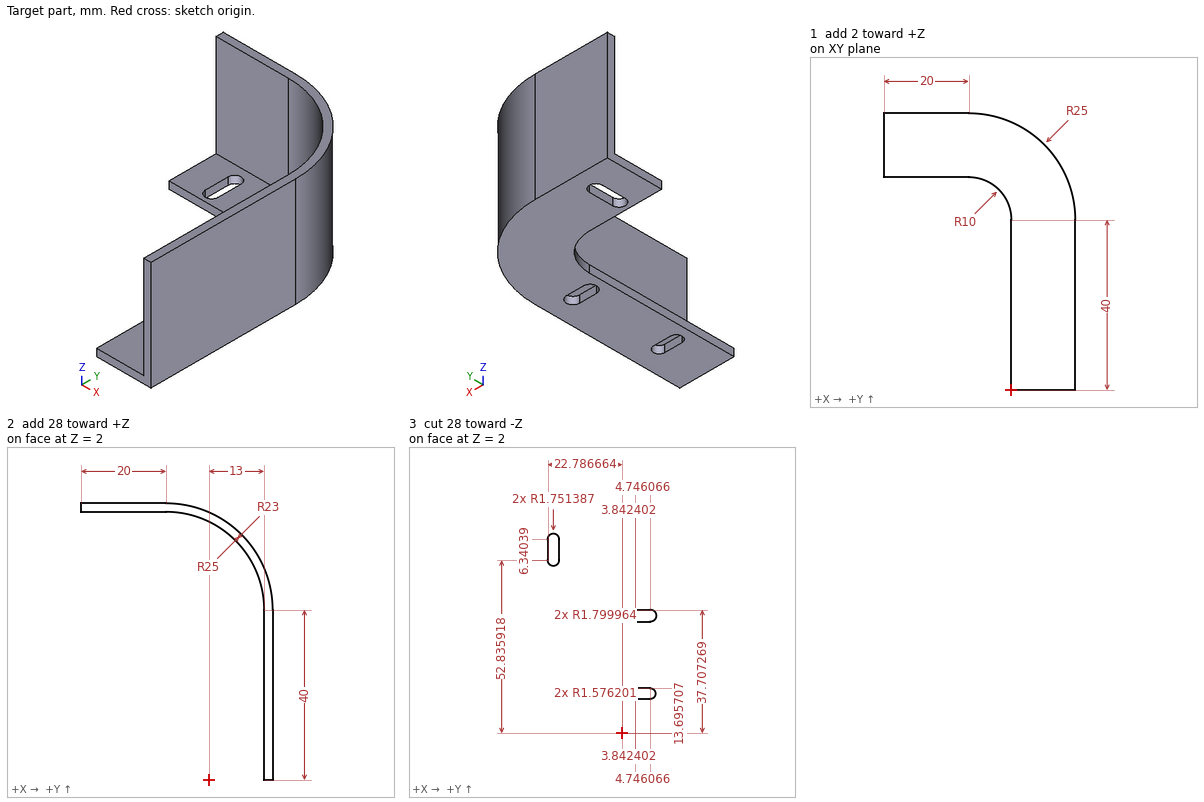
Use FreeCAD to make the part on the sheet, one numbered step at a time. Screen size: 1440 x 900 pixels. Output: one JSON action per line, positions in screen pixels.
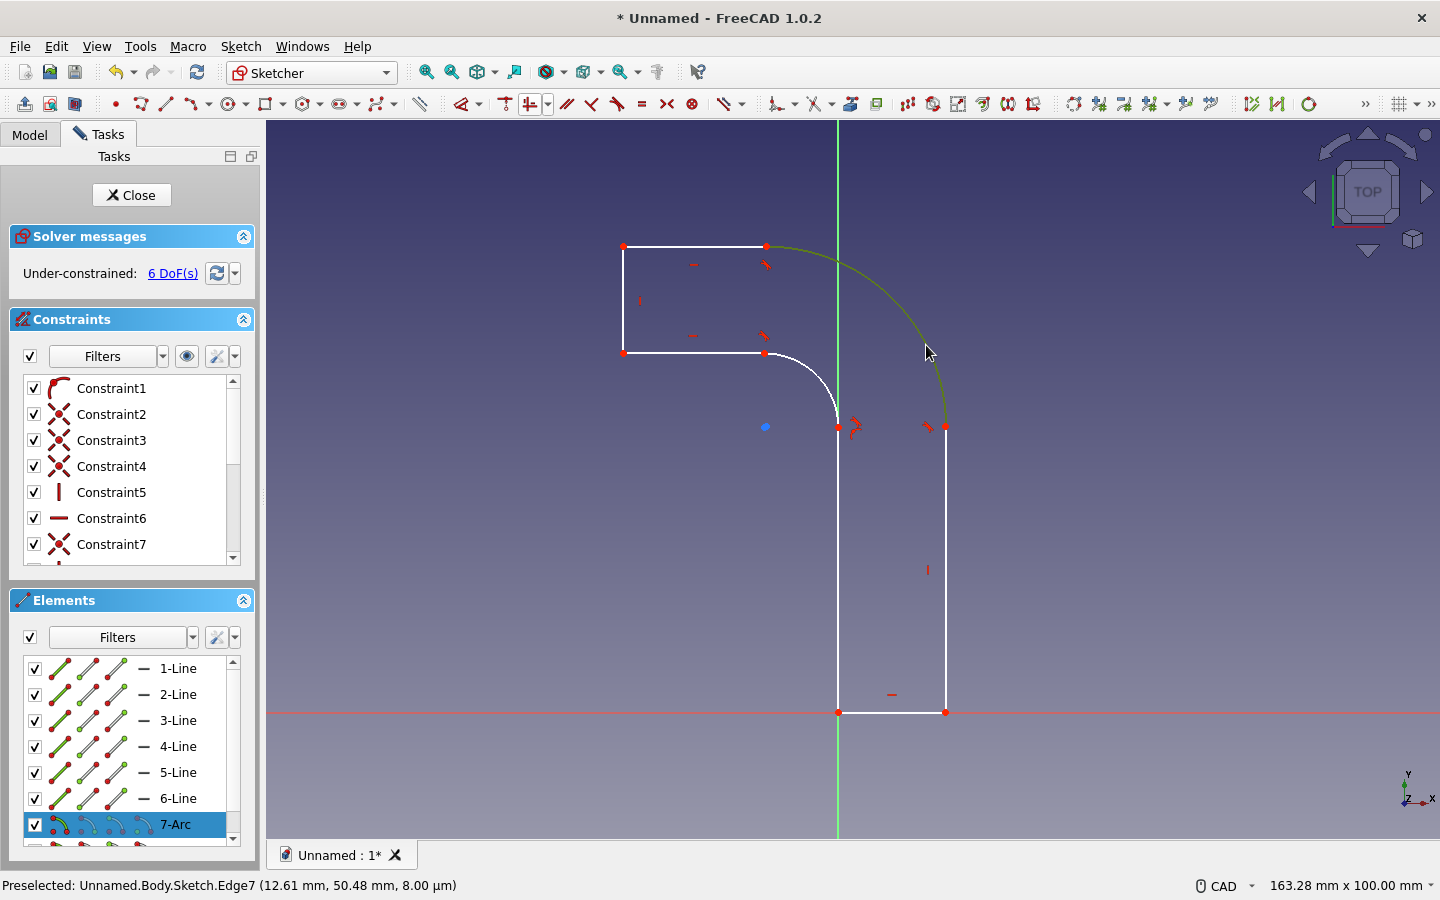
{"action": "left_click", "coordinate": [798, 362]}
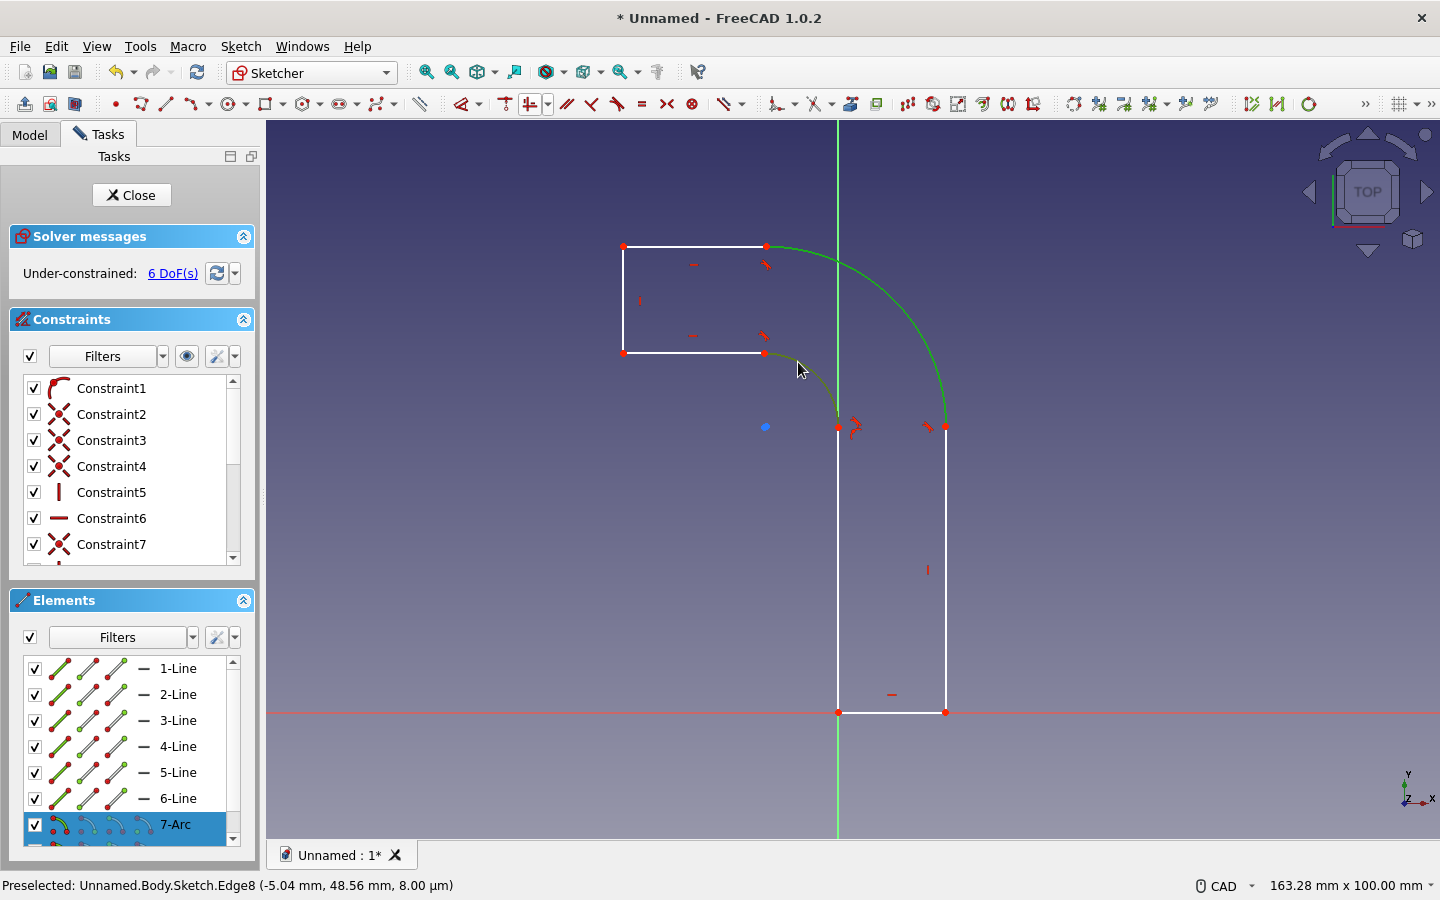
{"action": "left_click", "coordinate": [505, 104]}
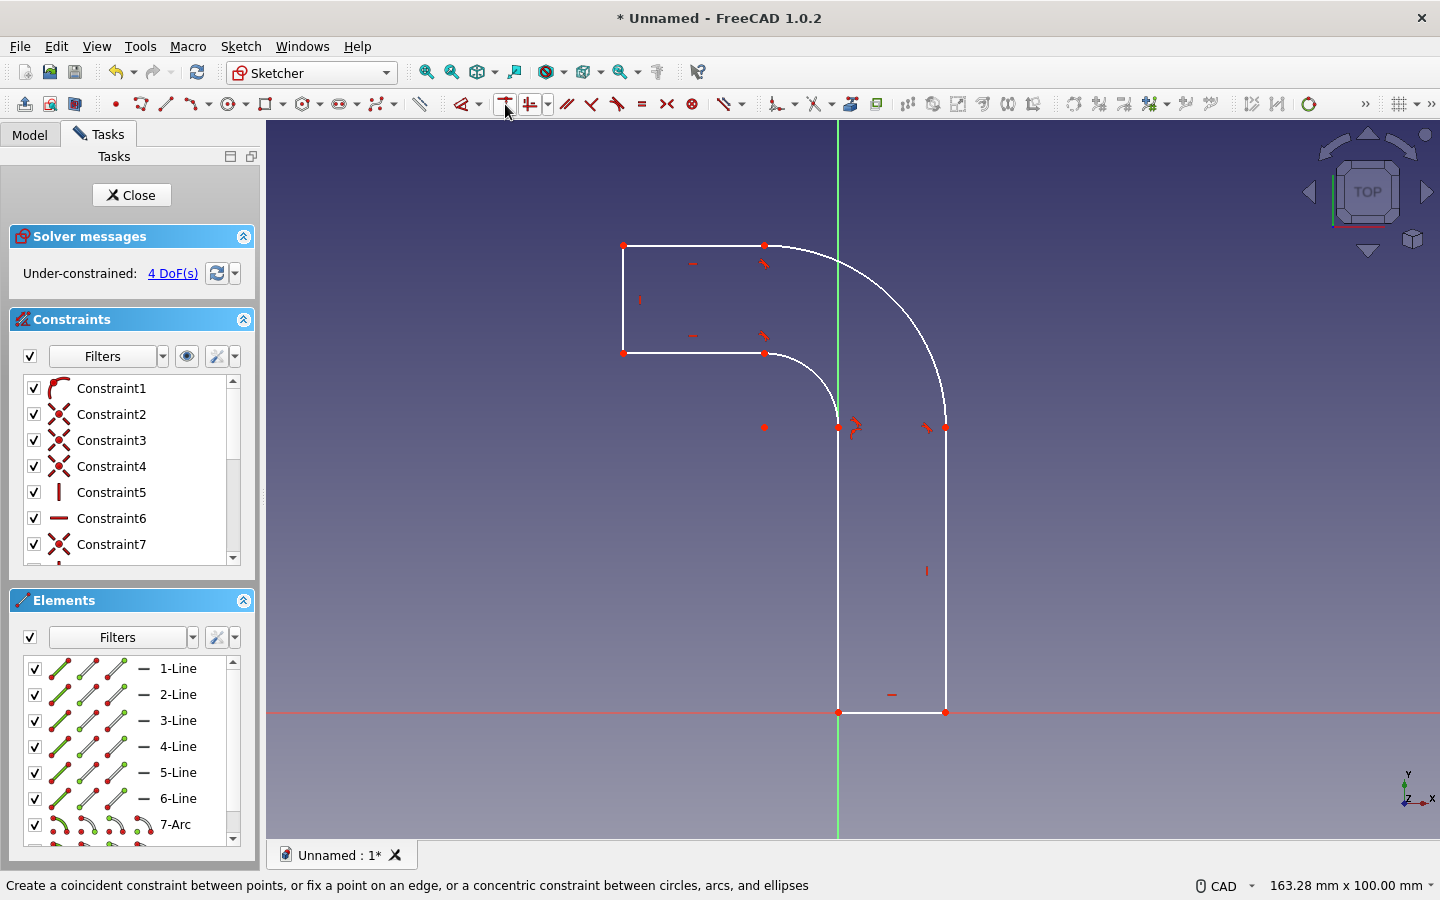
{"action": "left_click", "coordinate": [460, 104]}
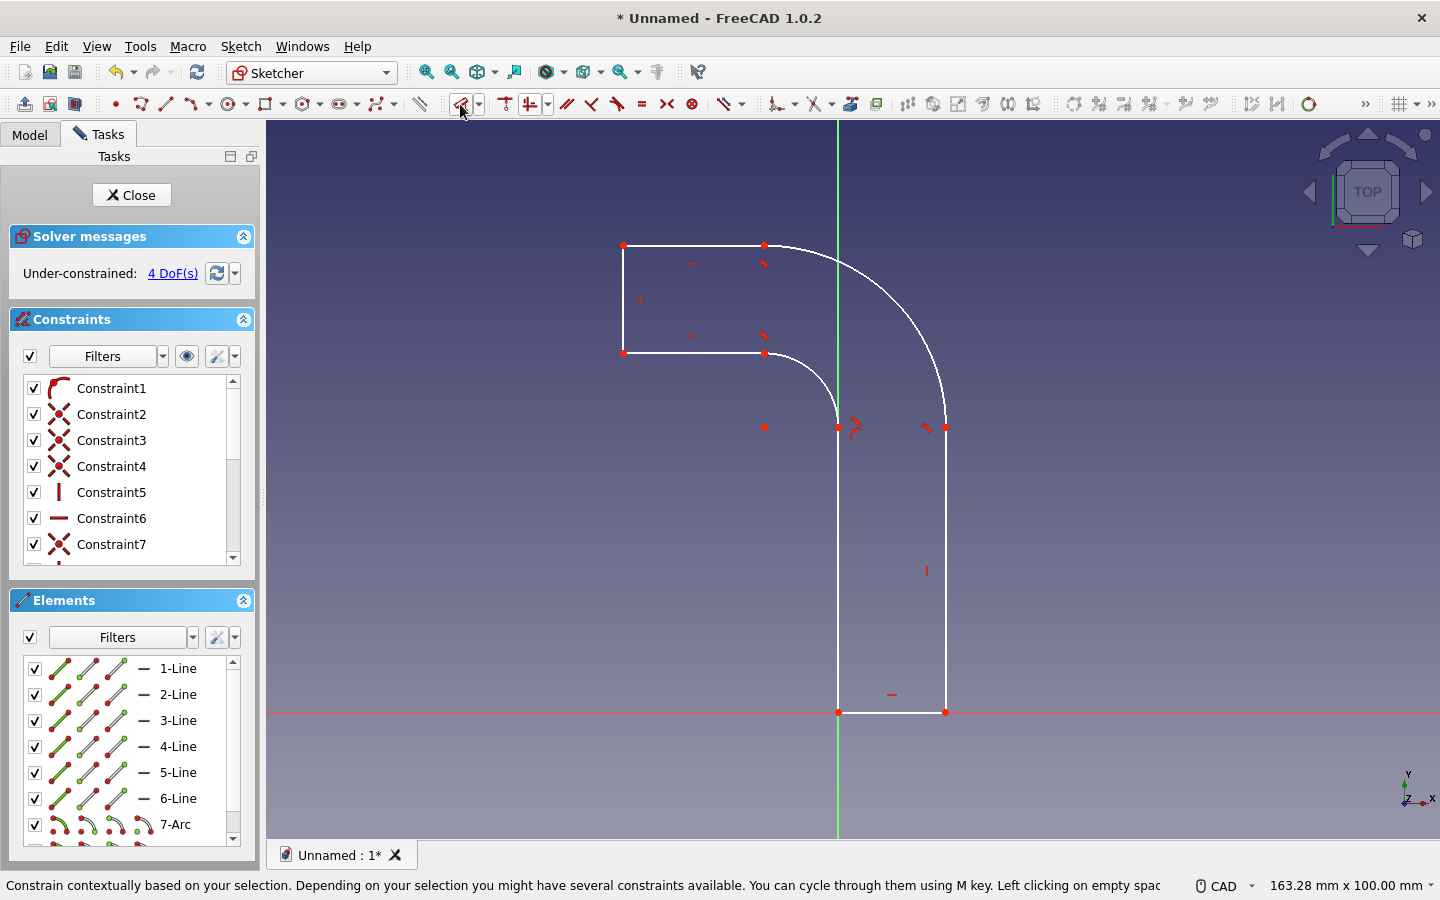
{"action": "left_click", "coordinate": [926, 345]}
{"action": "left_click", "coordinate": [955, 330]}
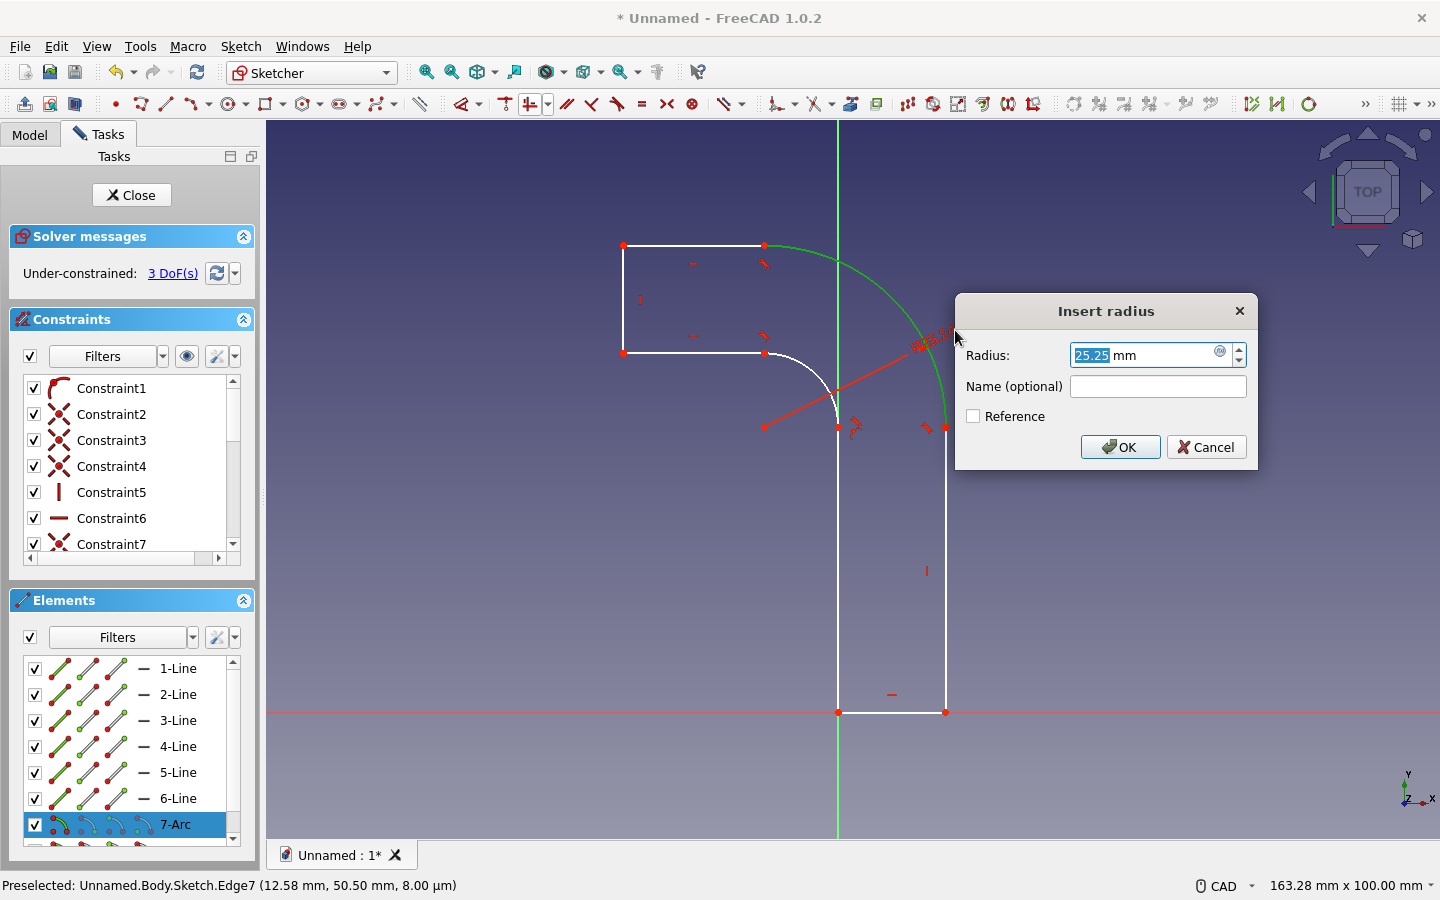
{"action": "type", "text": "25"}
{"action": "key", "text": "Return"}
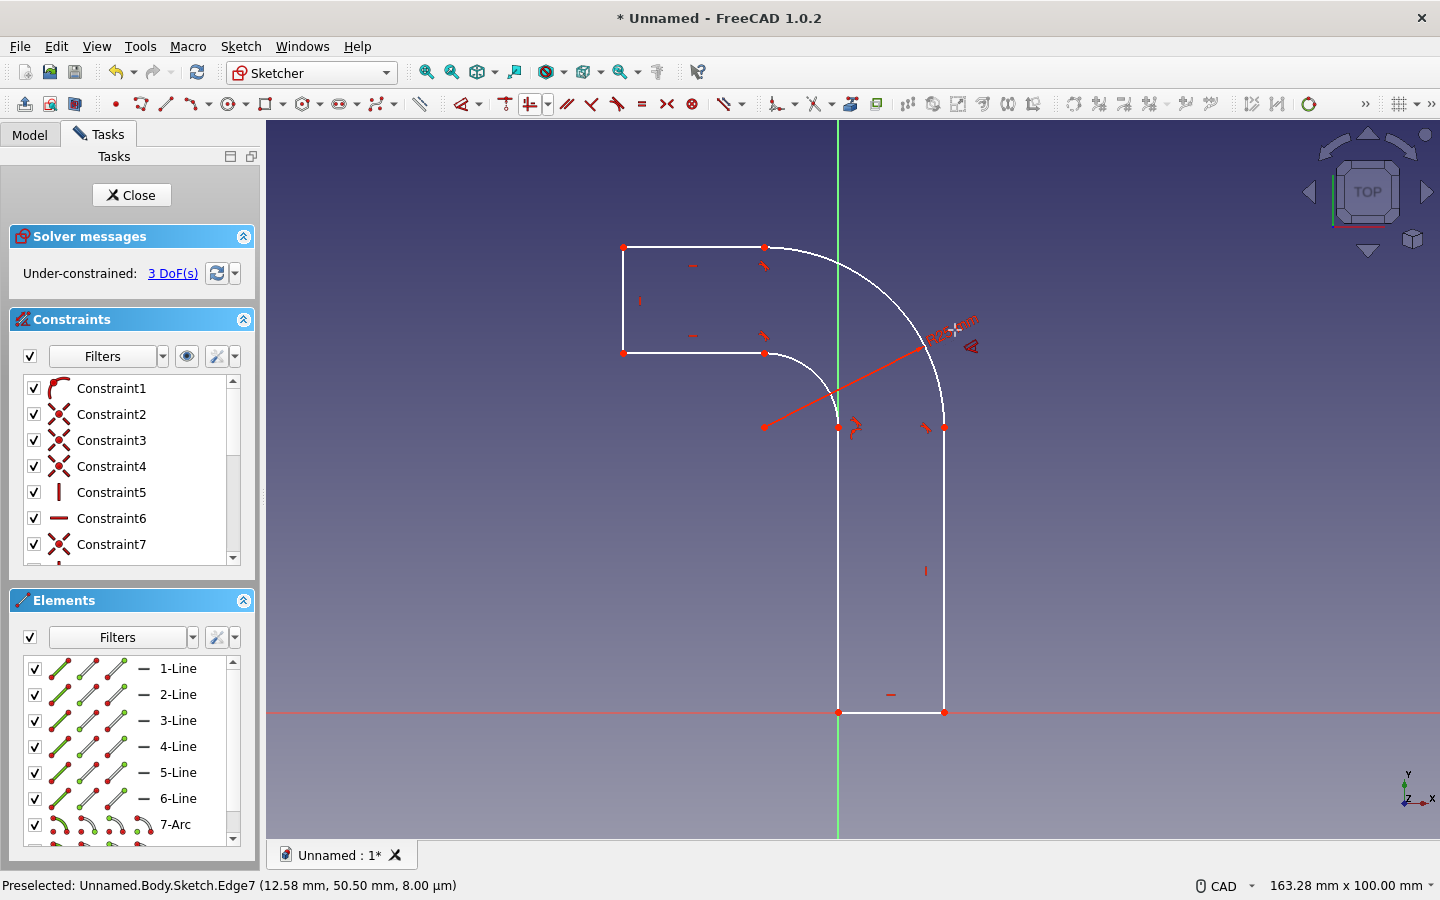
{"action": "left_click", "coordinate": [798, 361]}
{"action": "left_click", "coordinate": [812, 332]}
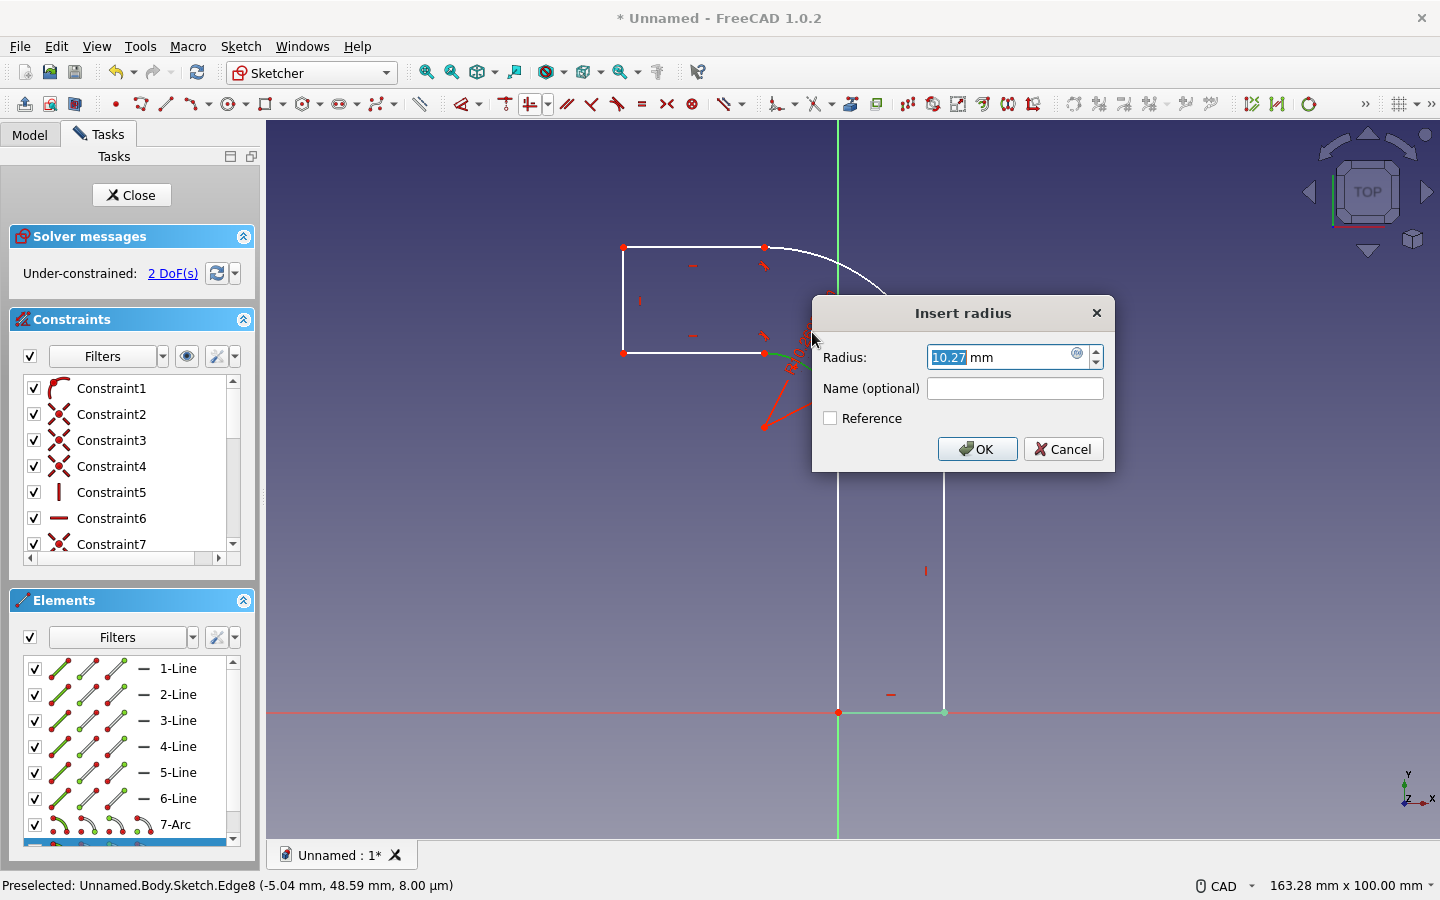
{"action": "type", "text": "10"}
{"action": "key", "text": "Return"}